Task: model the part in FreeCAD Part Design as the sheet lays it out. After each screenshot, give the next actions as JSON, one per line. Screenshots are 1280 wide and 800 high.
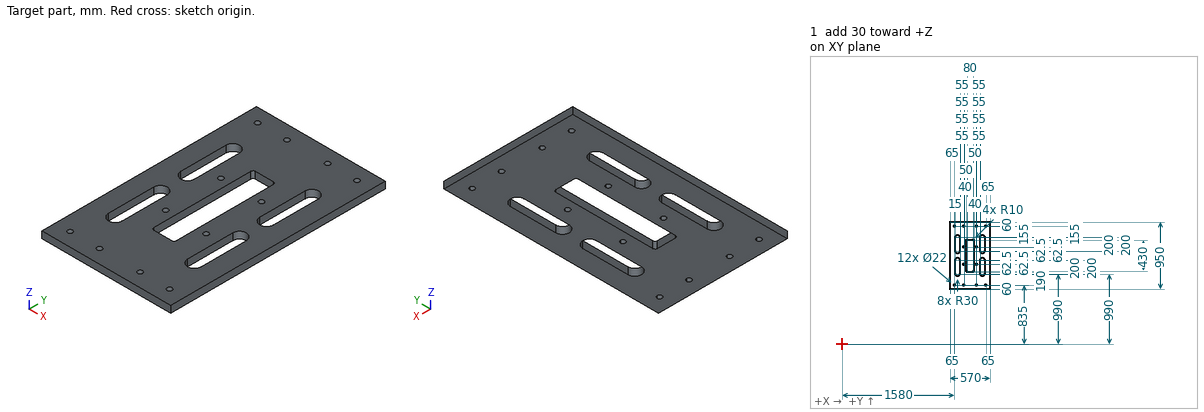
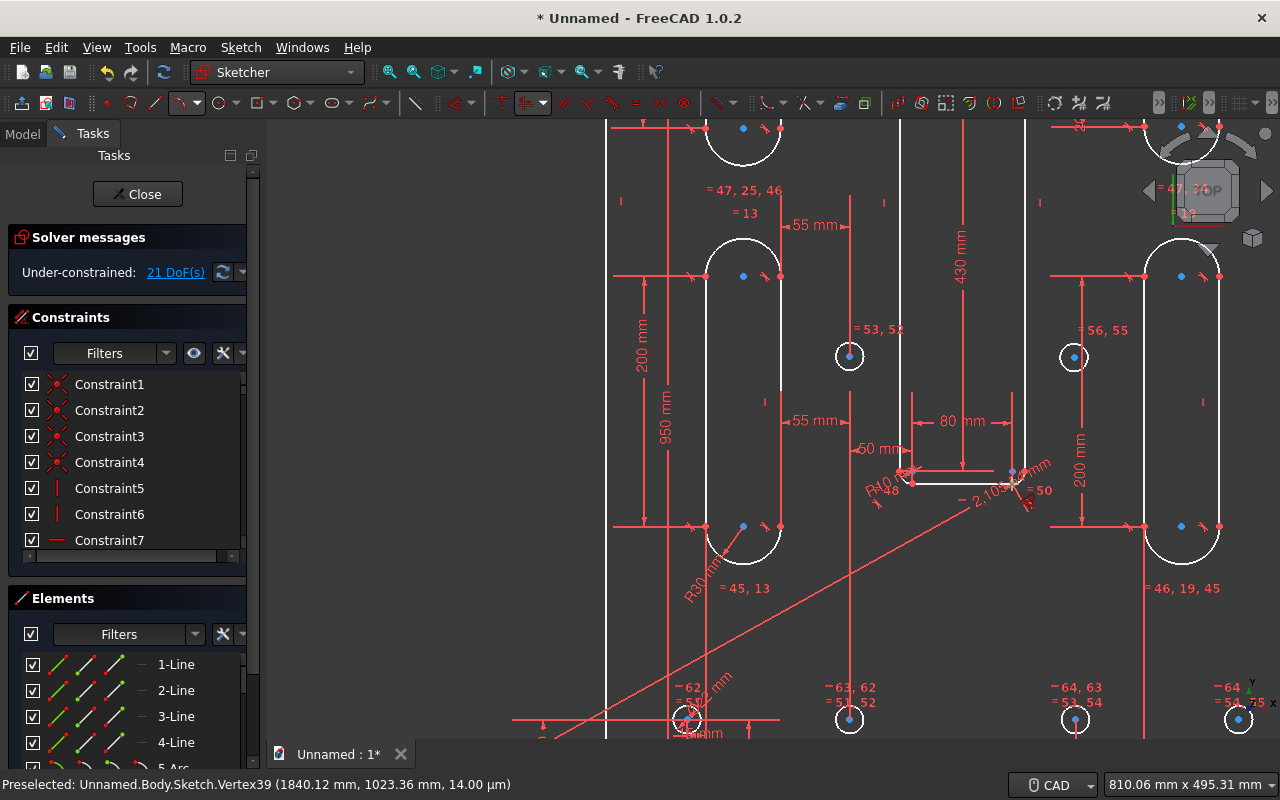
{"action": "scroll", "coordinate": [879, 364], "scroll_direction": "down", "scroll_amount": 8}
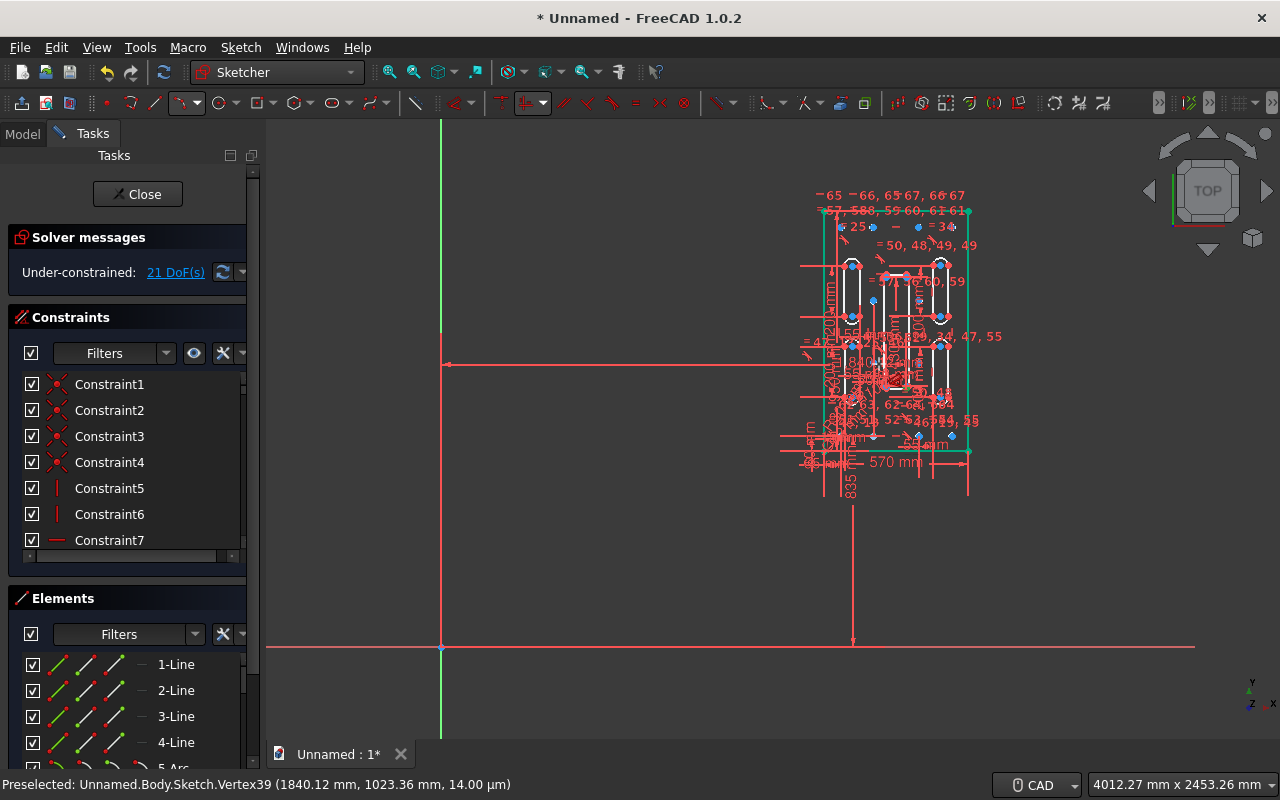
{"action": "scroll", "coordinate": [919, 436], "scroll_direction": "up", "scroll_amount": 6}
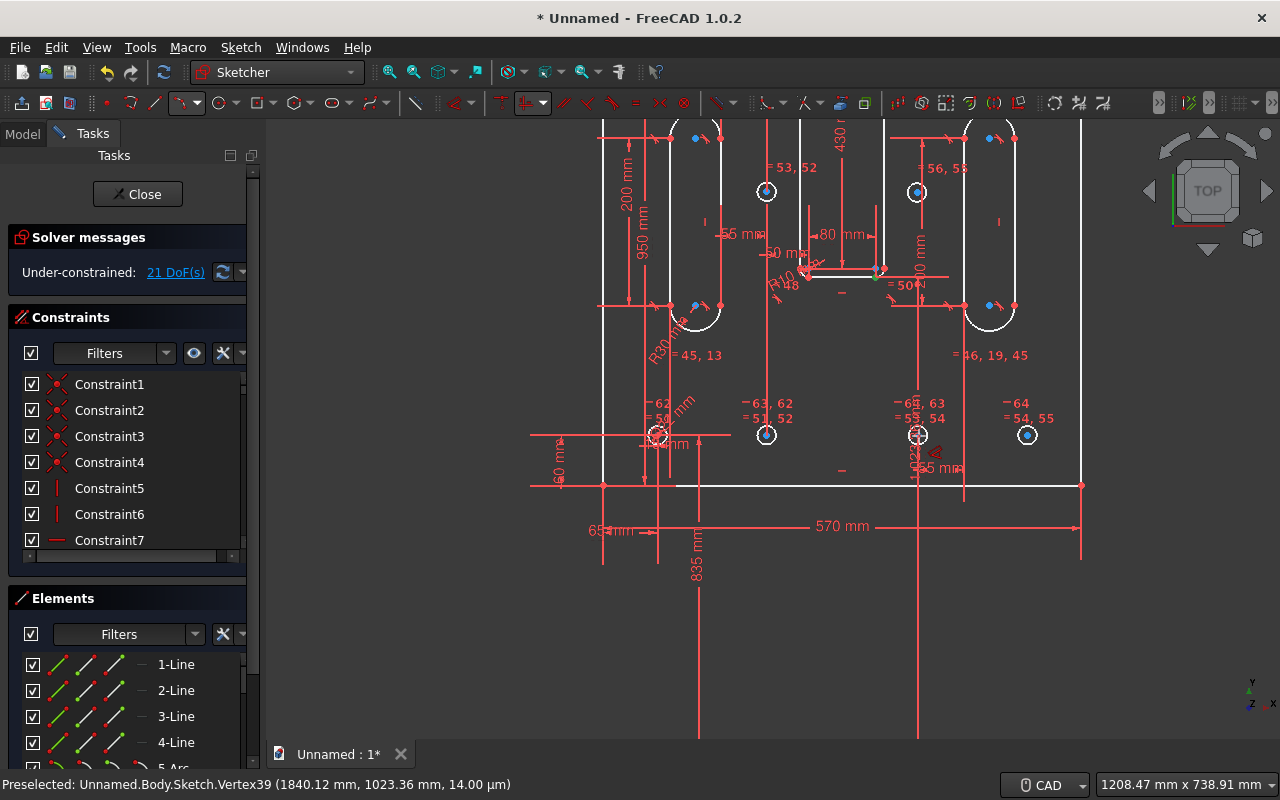
{"action": "left_click", "coordinate": [918, 435]}
{"action": "left_click", "coordinate": [912, 517]}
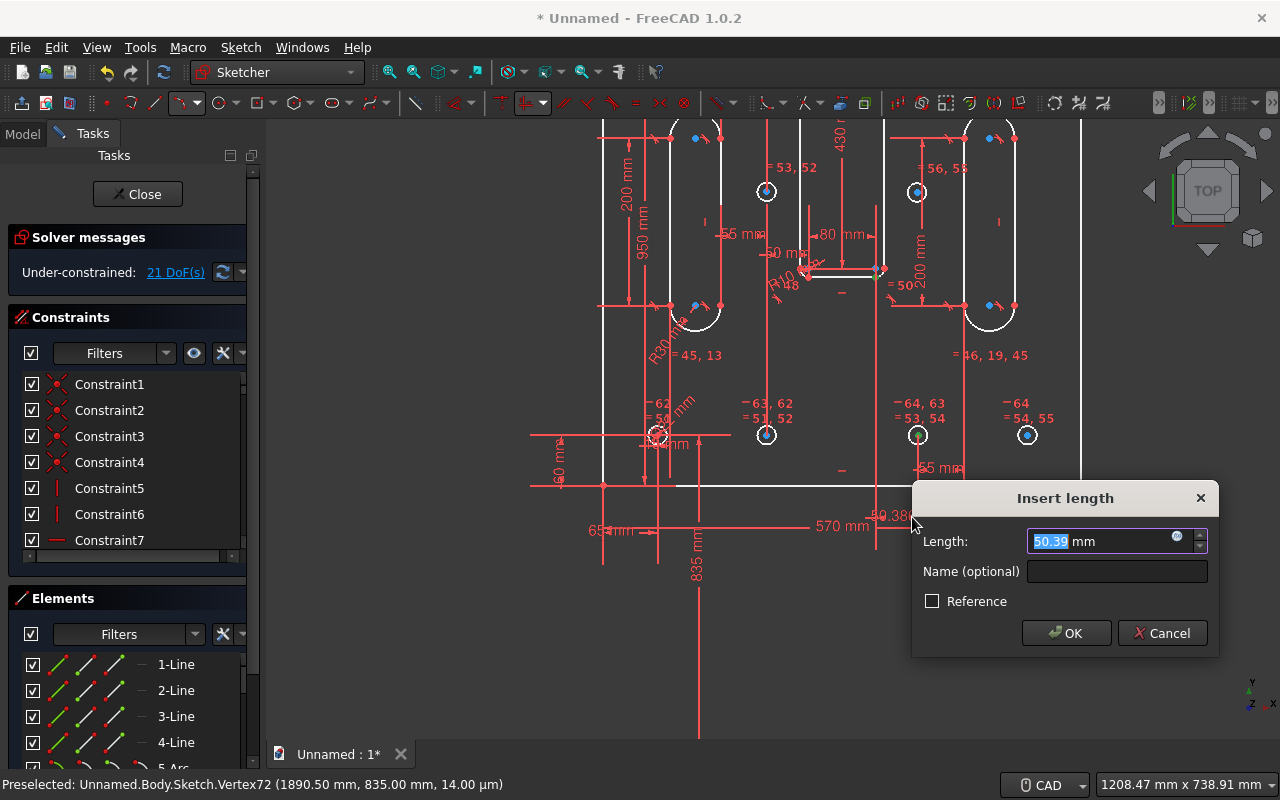
{"action": "type", "text": "50"}
{"action": "key", "text": "Return"}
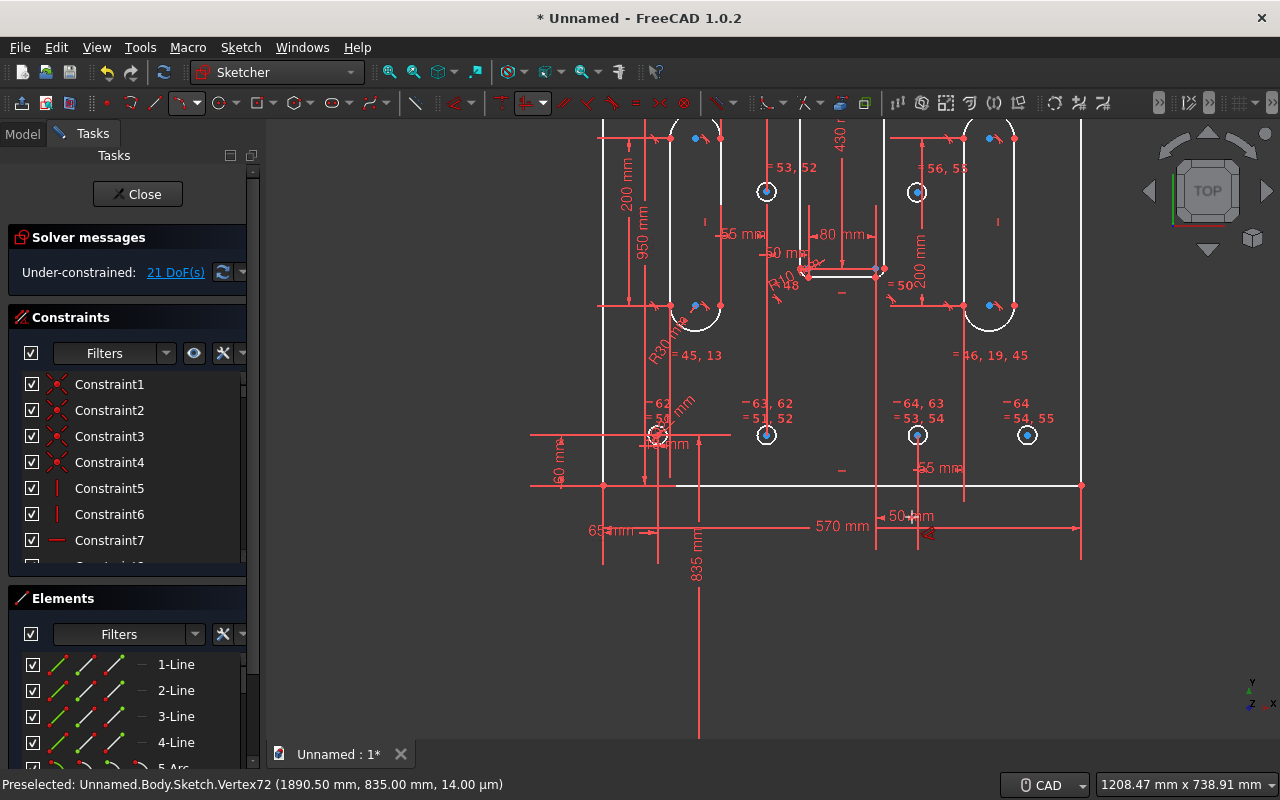
{"action": "left_click", "coordinate": [1081, 486]}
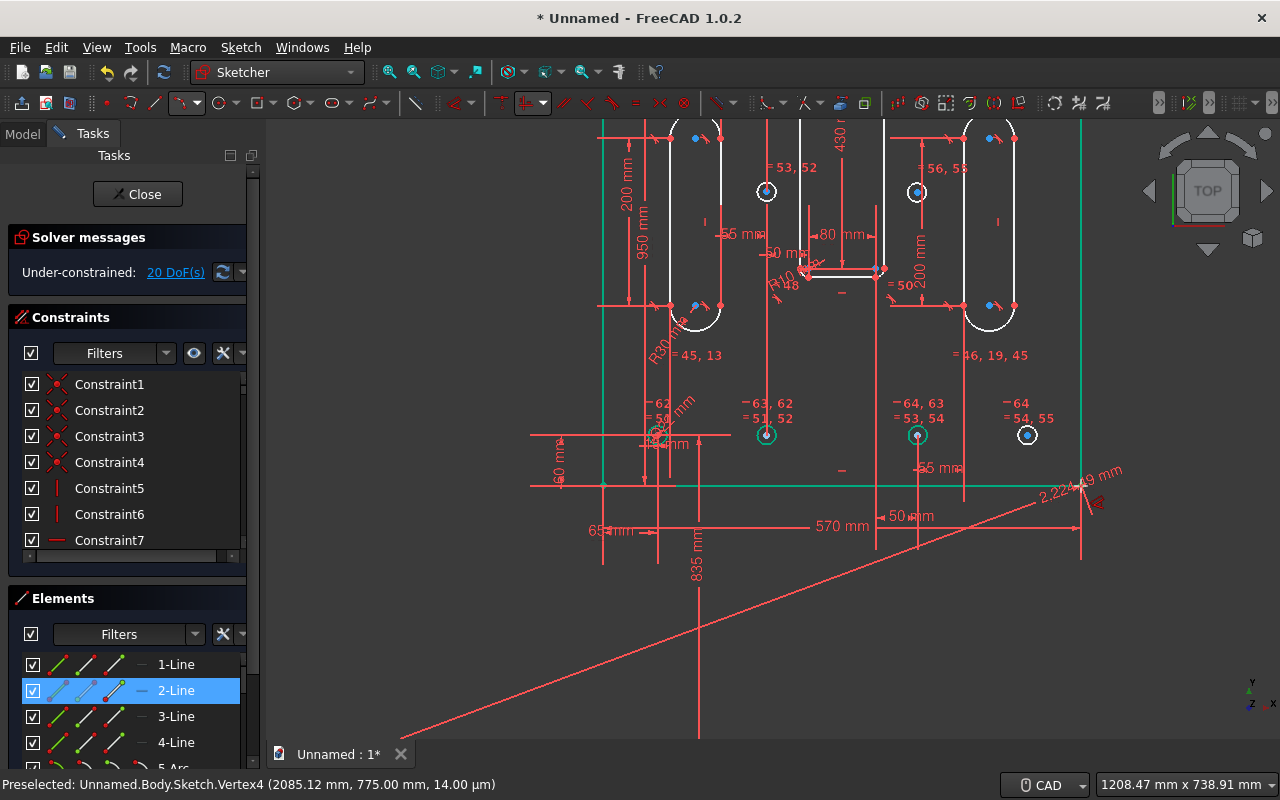
{"action": "left_click", "coordinate": [1027, 435]}
{"action": "left_click", "coordinate": [1054, 520]}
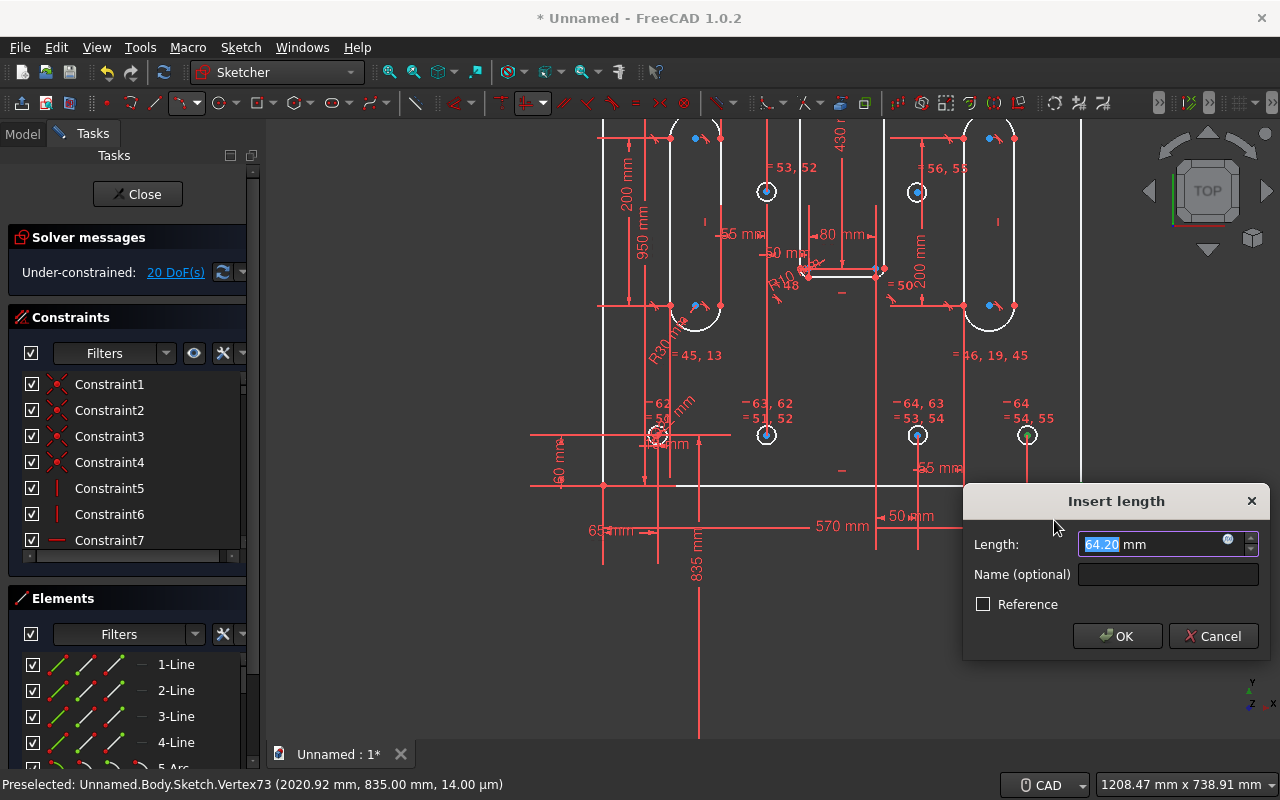
{"action": "type", "text": "65"}
{"action": "key", "text": "Return"}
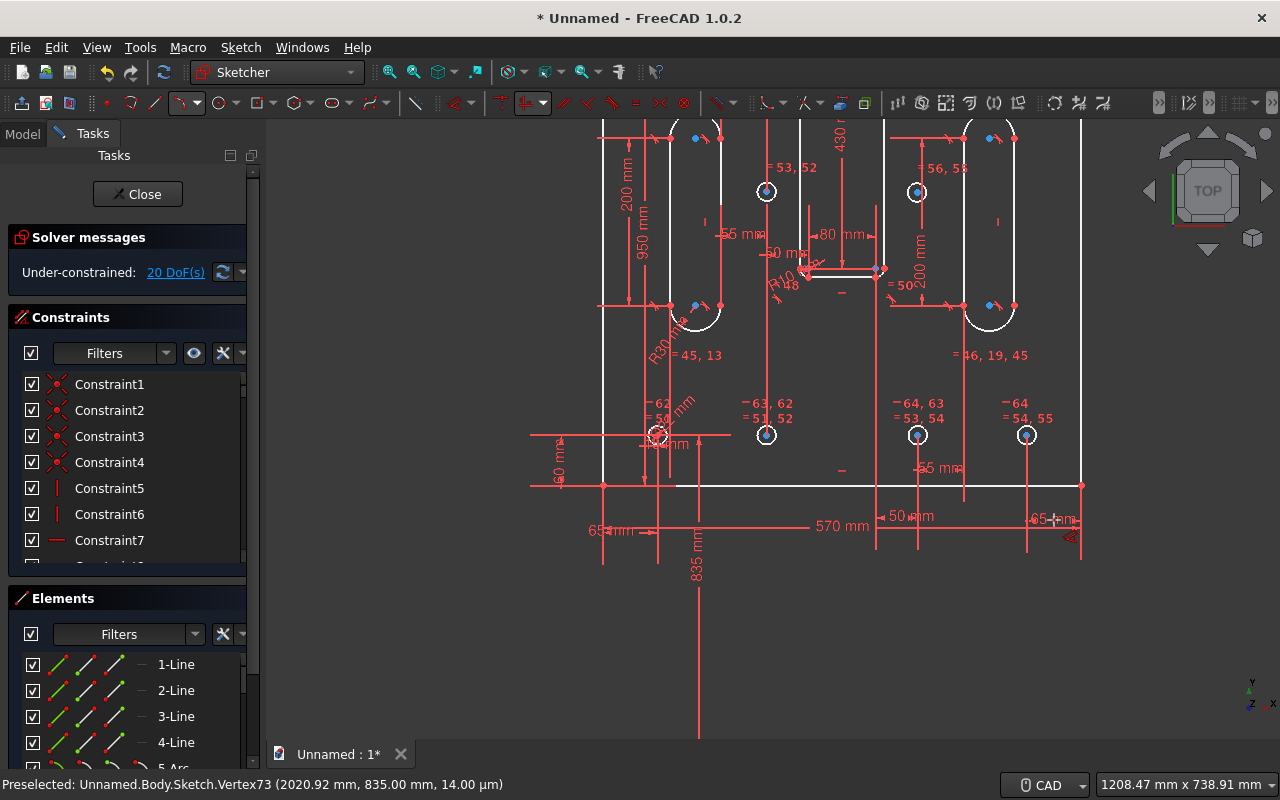
{"action": "scroll", "coordinate": [919, 436], "scroll_direction": "down", "scroll_amount": 6}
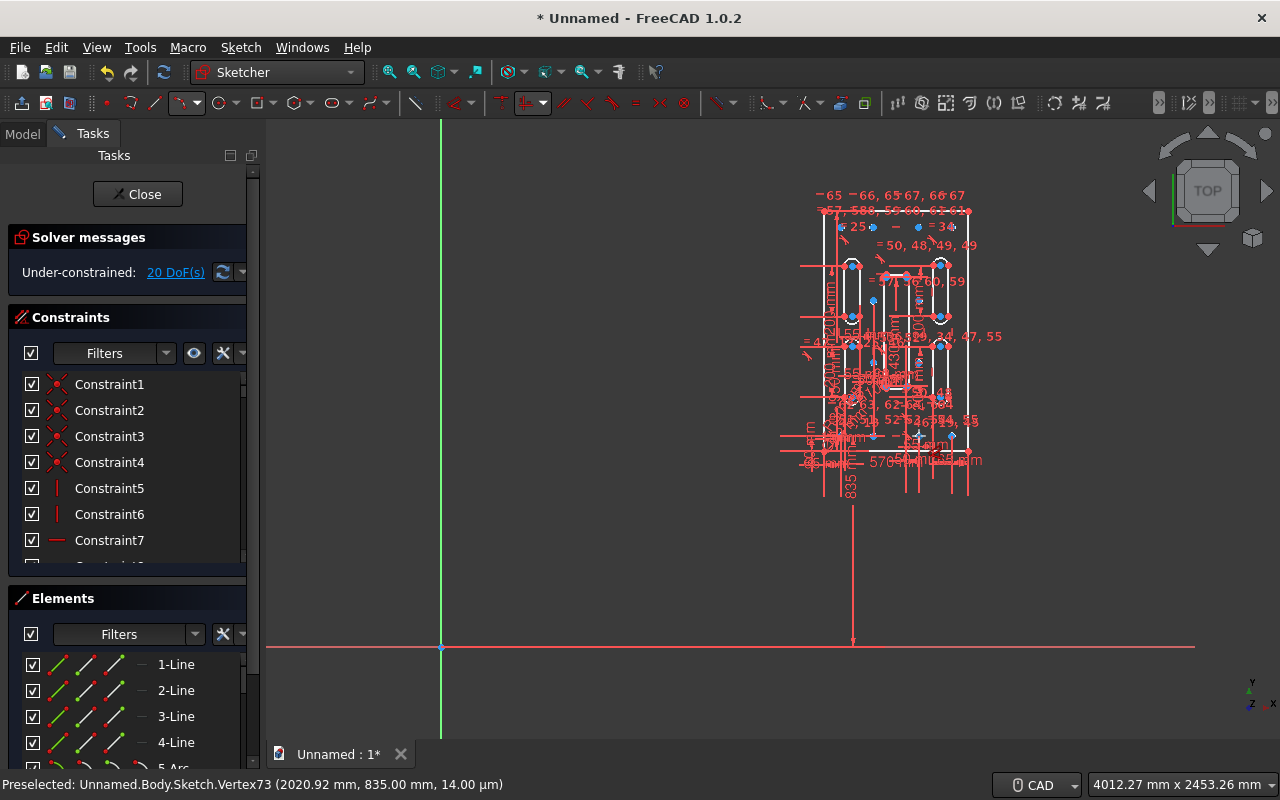
{"action": "scroll", "coordinate": [933, 347], "scroll_direction": "up", "scroll_amount": 6}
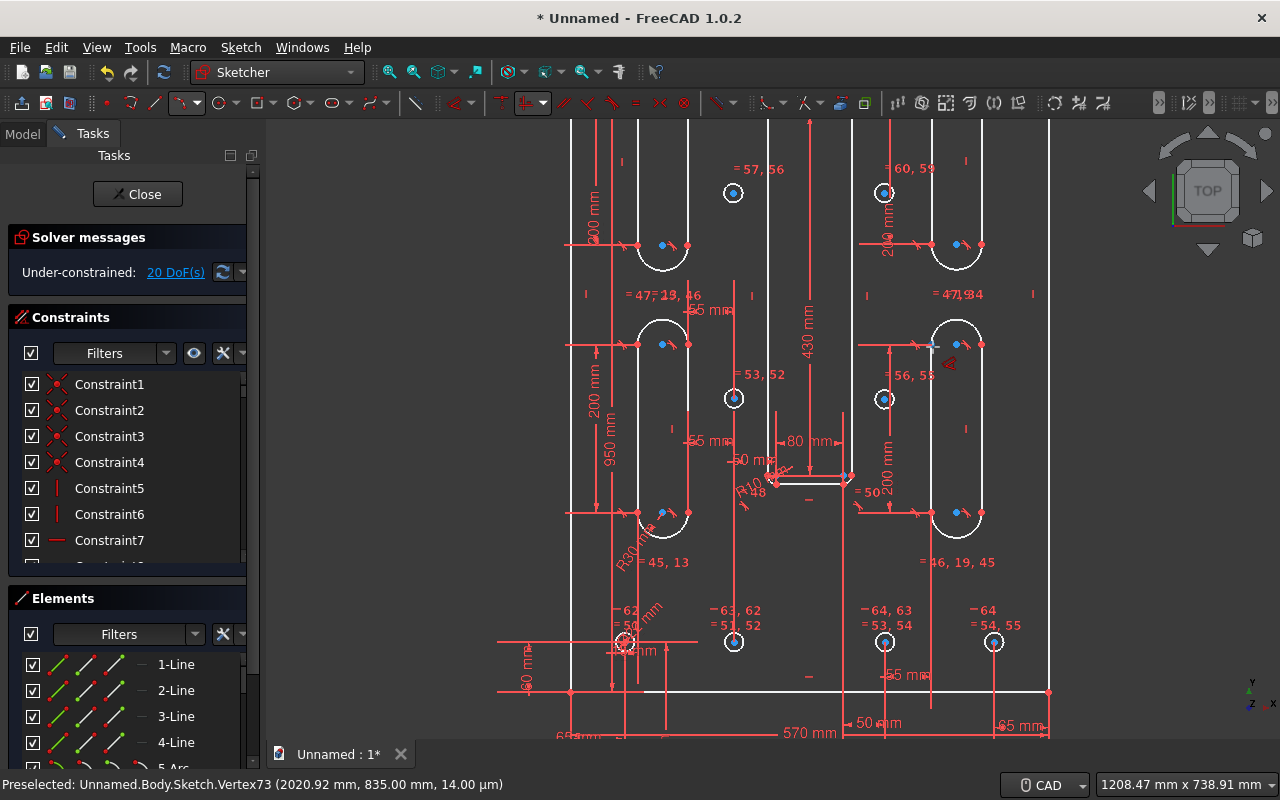
{"action": "left_click", "coordinate": [931, 345]}